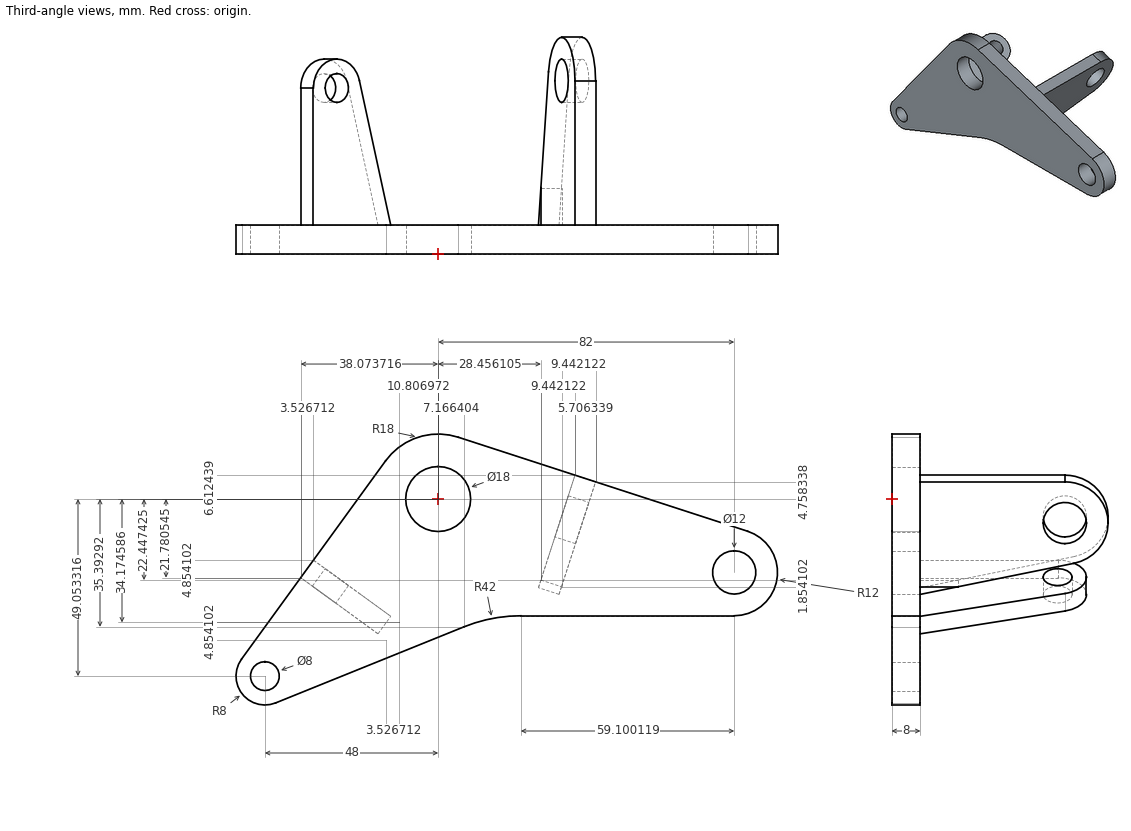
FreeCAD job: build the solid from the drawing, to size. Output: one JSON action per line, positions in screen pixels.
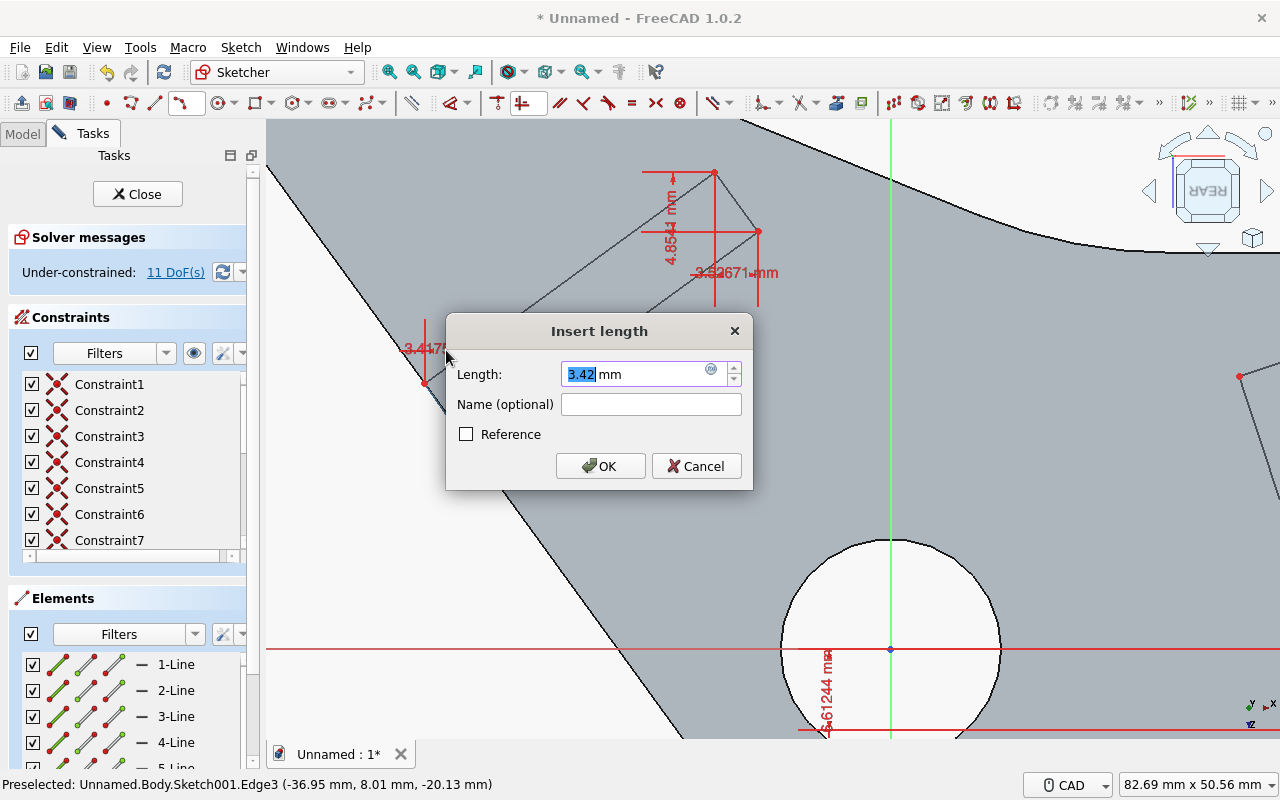
{"action": "type", "text": "3.526712"}
{"action": "key", "text": "Return"}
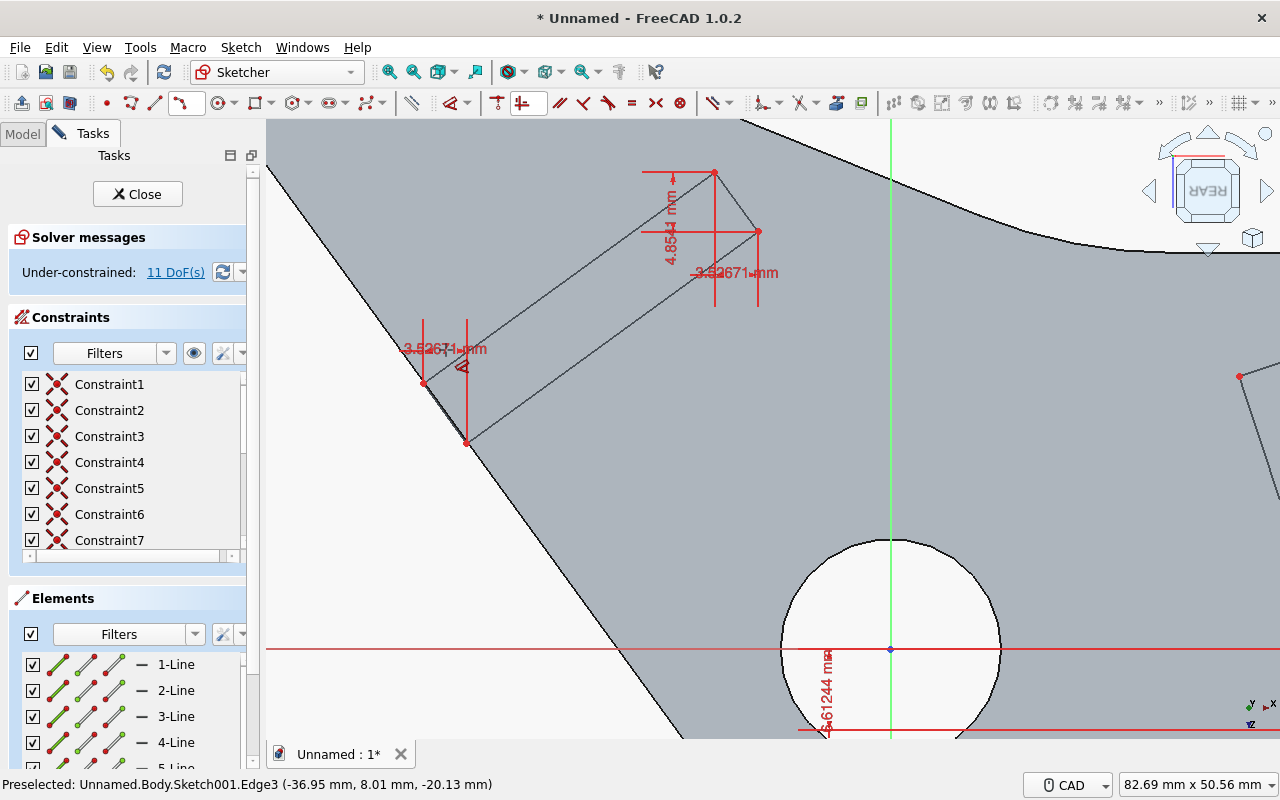
{"action": "left_click", "coordinate": [436, 402]}
{"action": "left_click", "coordinate": [389, 414]}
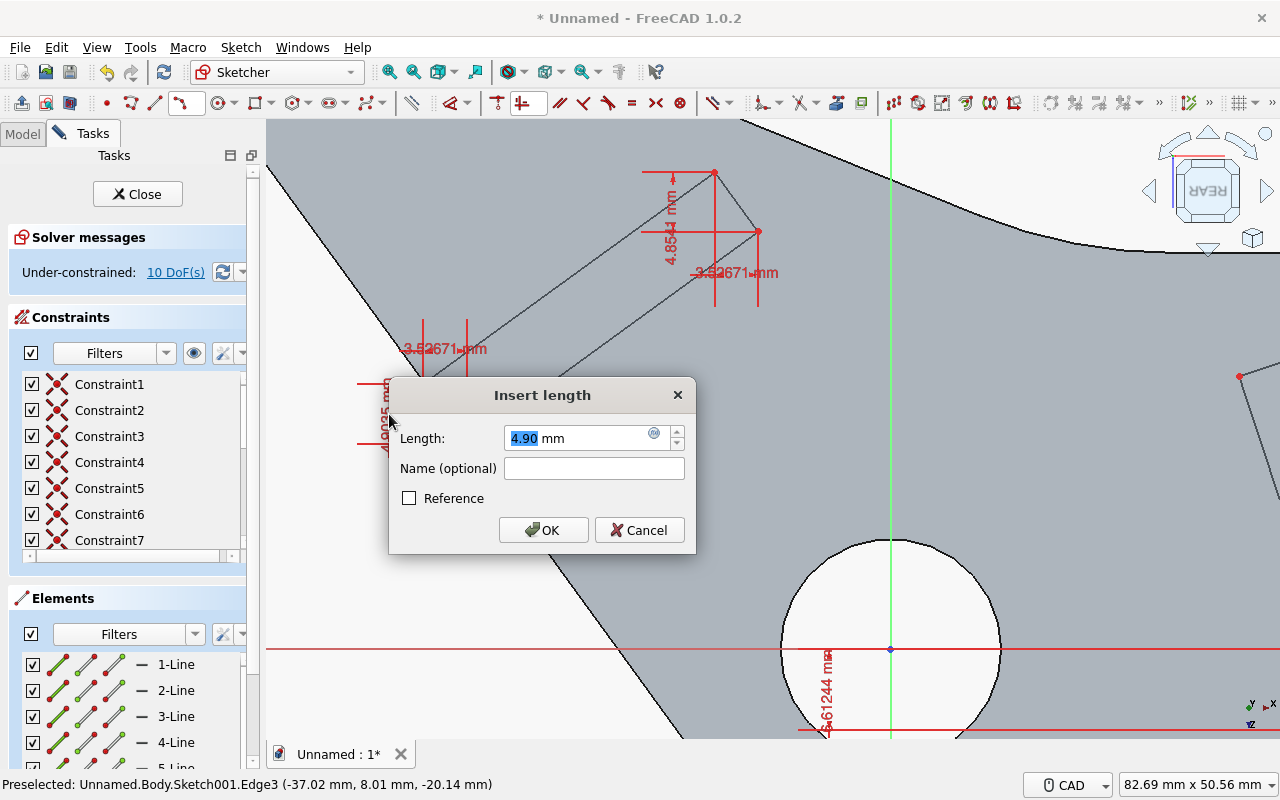
{"action": "type", "text": "4.854102"}
{"action": "key", "text": "Return"}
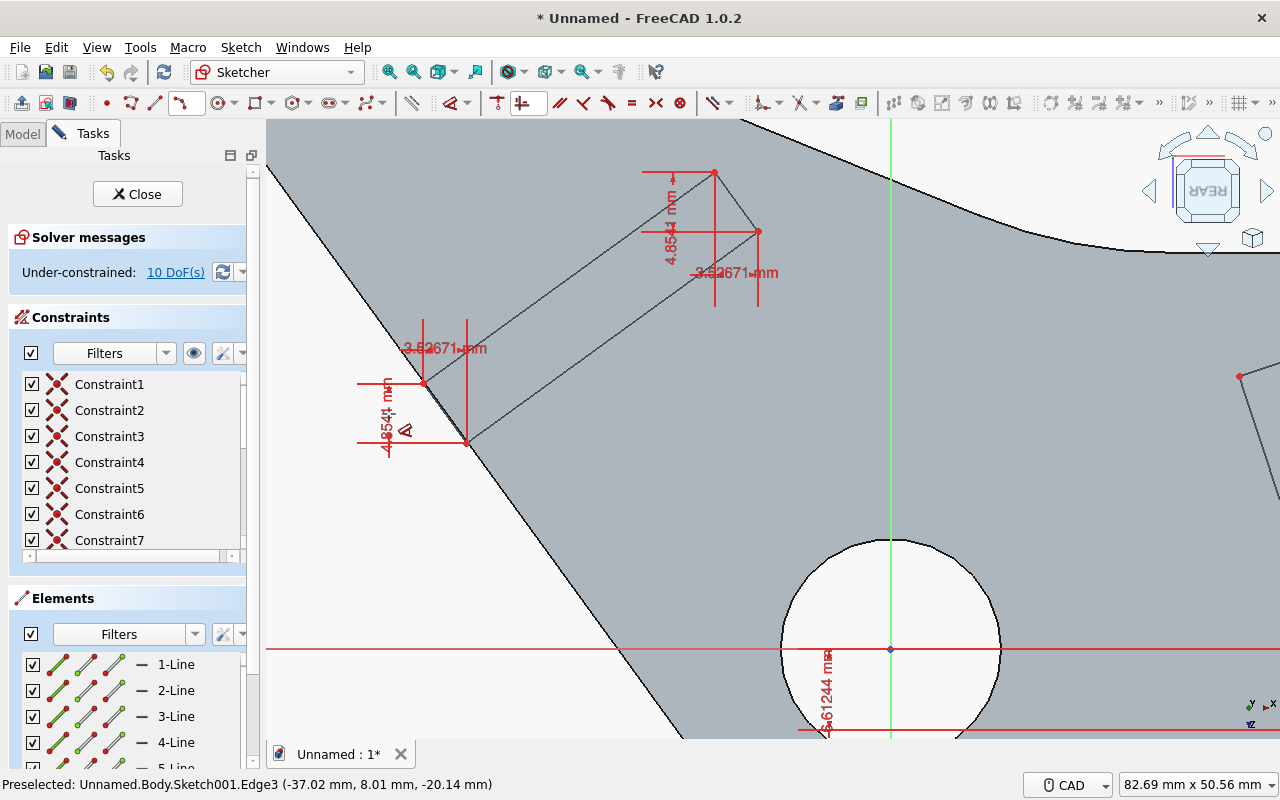
{"action": "scroll", "coordinate": [437, 403], "scroll_direction": "down", "scroll_amount": 3}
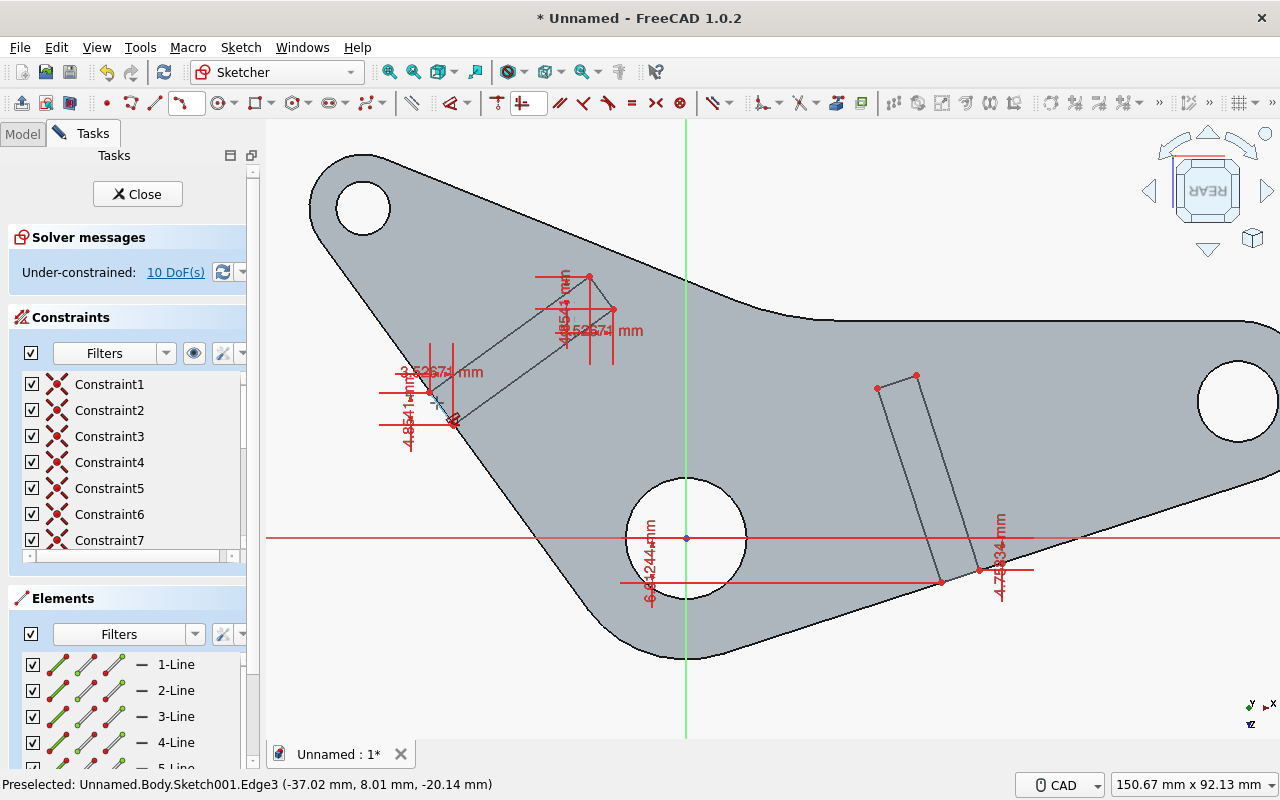
{"action": "left_click", "coordinate": [897, 447]}
{"action": "left_click", "coordinate": [909, 617]}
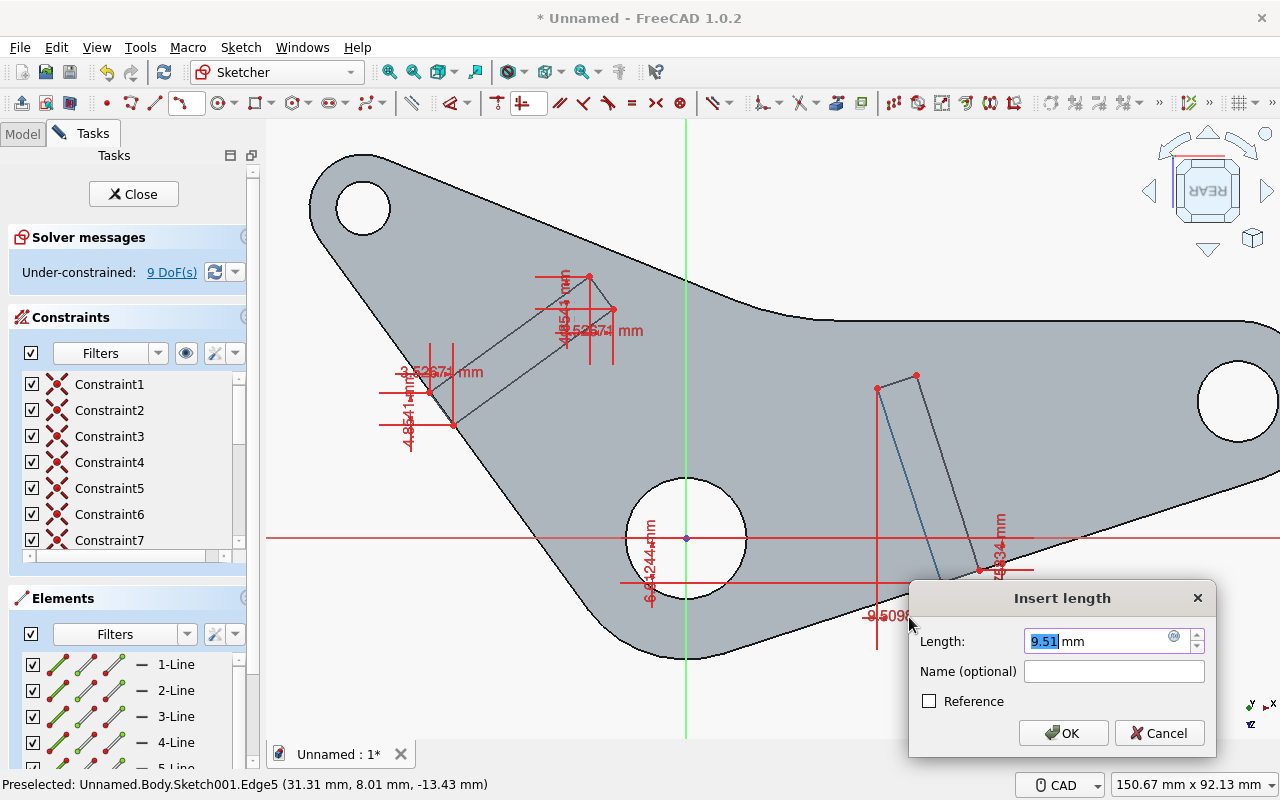
{"action": "type", "text": "9.442122"}
{"action": "key", "text": "Return"}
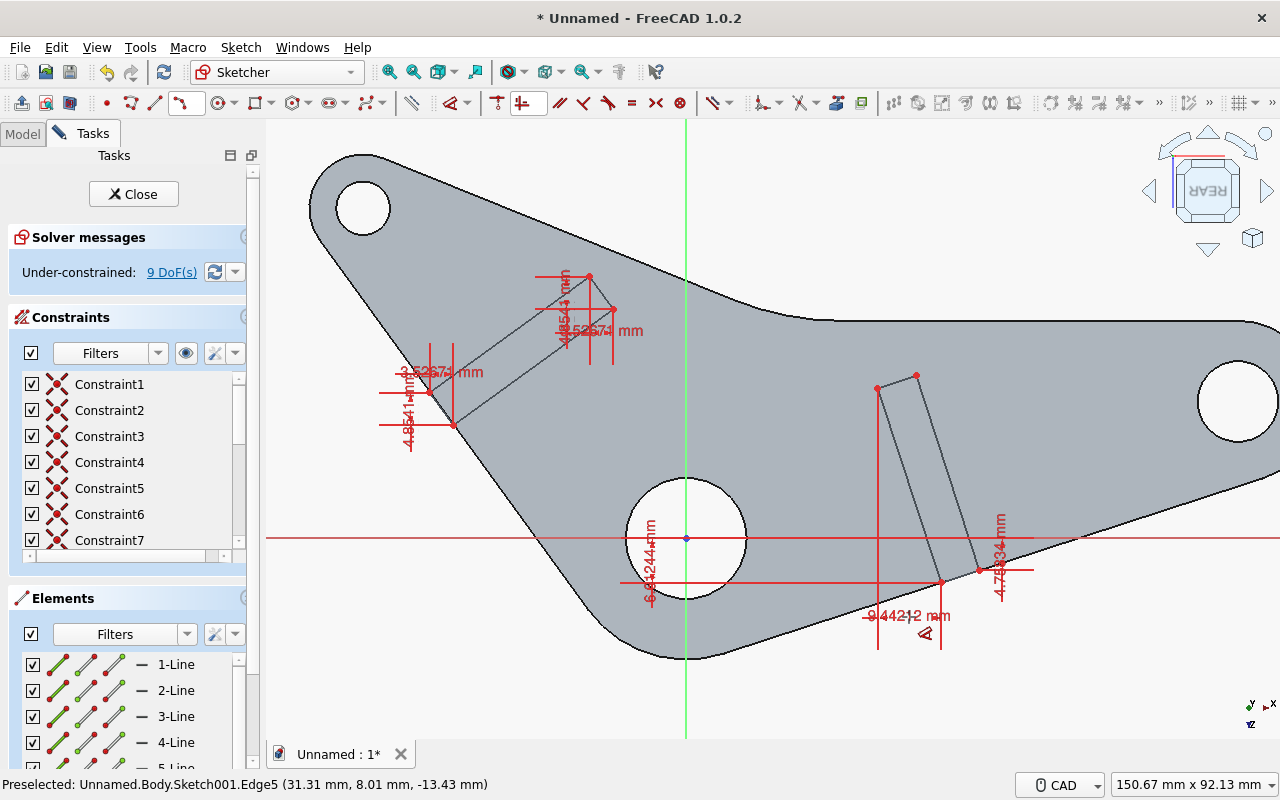
{"action": "left_click", "coordinate": [953, 579]}
{"action": "left_click", "coordinate": [960, 641]}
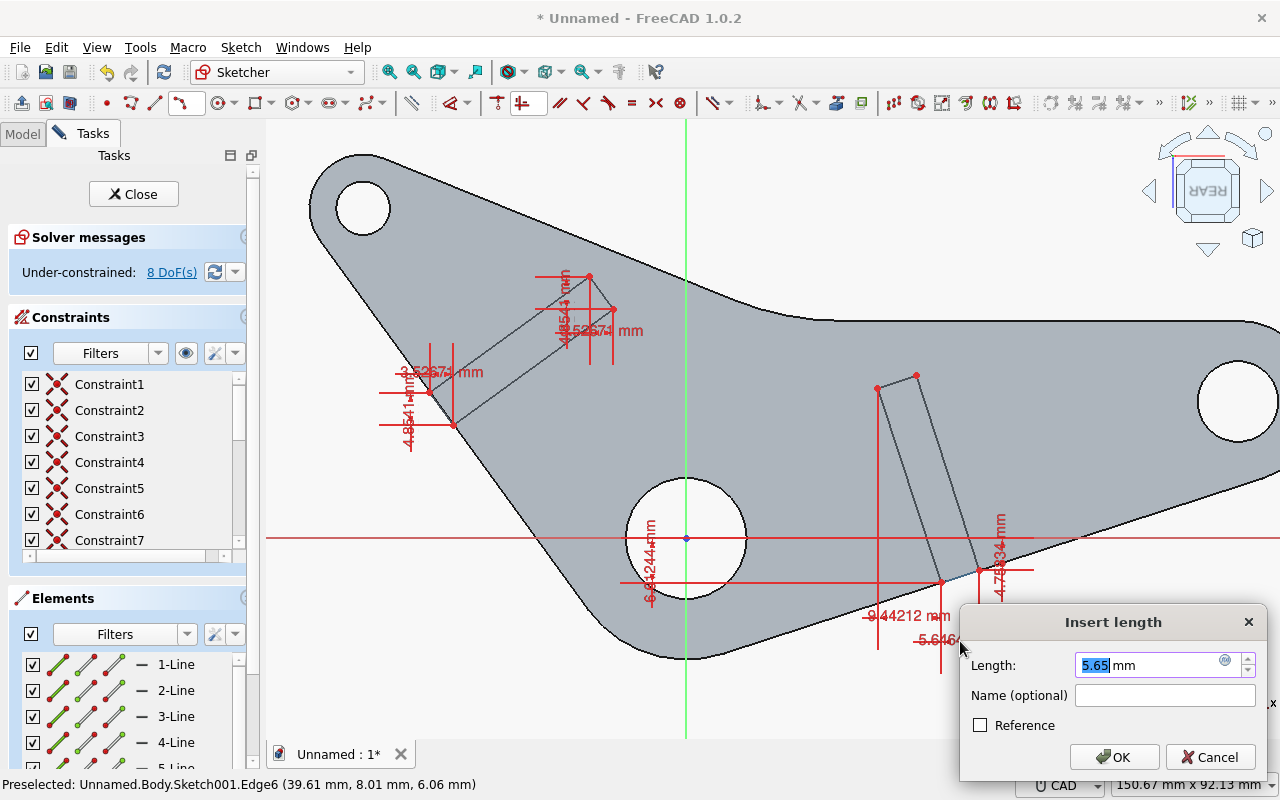
{"action": "type", "text": "5.706339"}
{"action": "key", "text": "Return"}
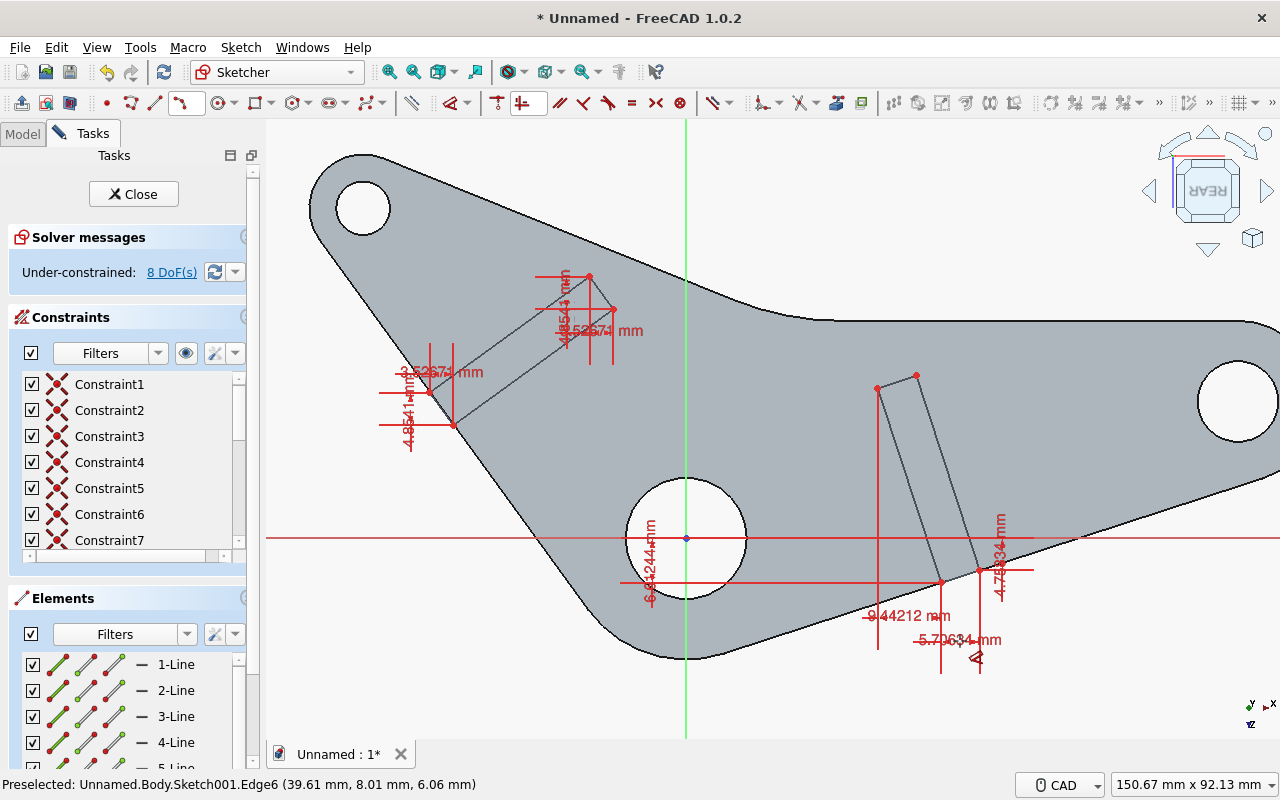
{"action": "left_click", "coordinate": [961, 512]}
{"action": "left_click", "coordinate": [948, 342]}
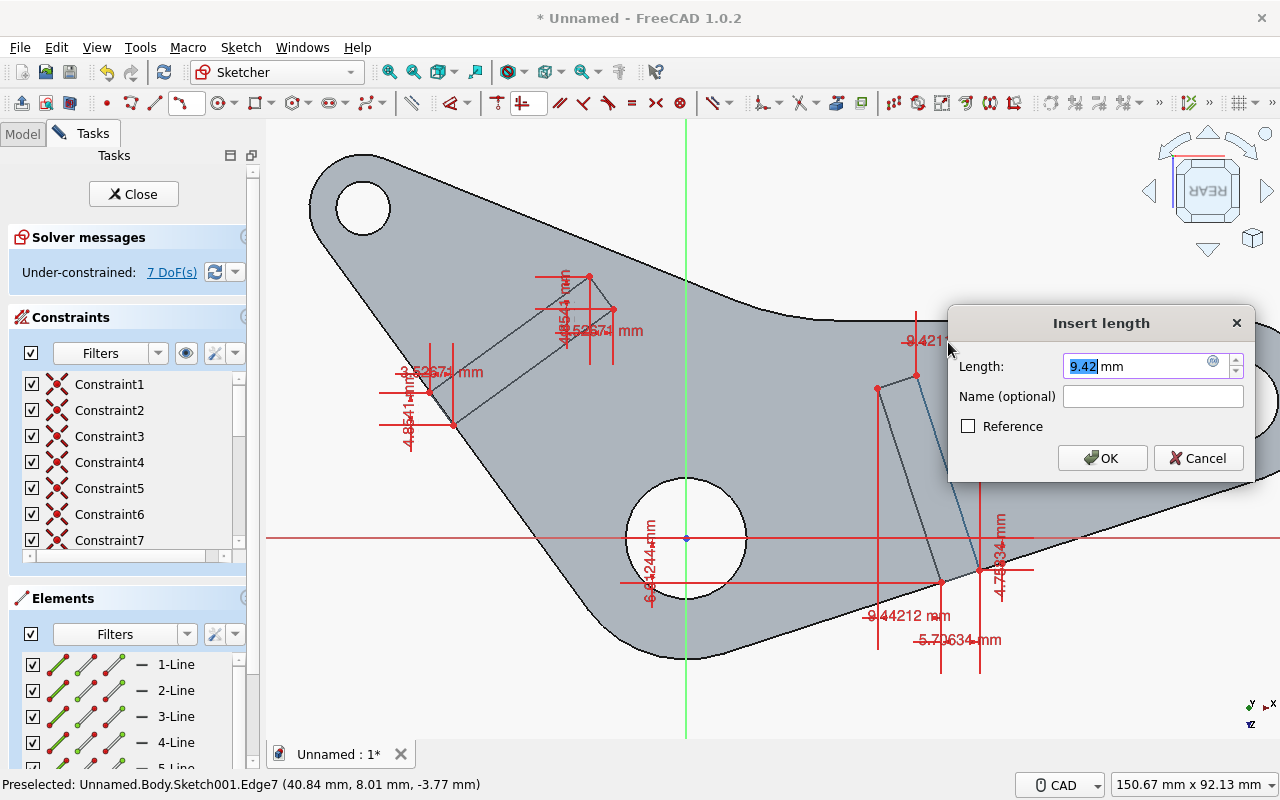
{"action": "type", "text": "9.442122"}
{"action": "key", "text": "Return"}